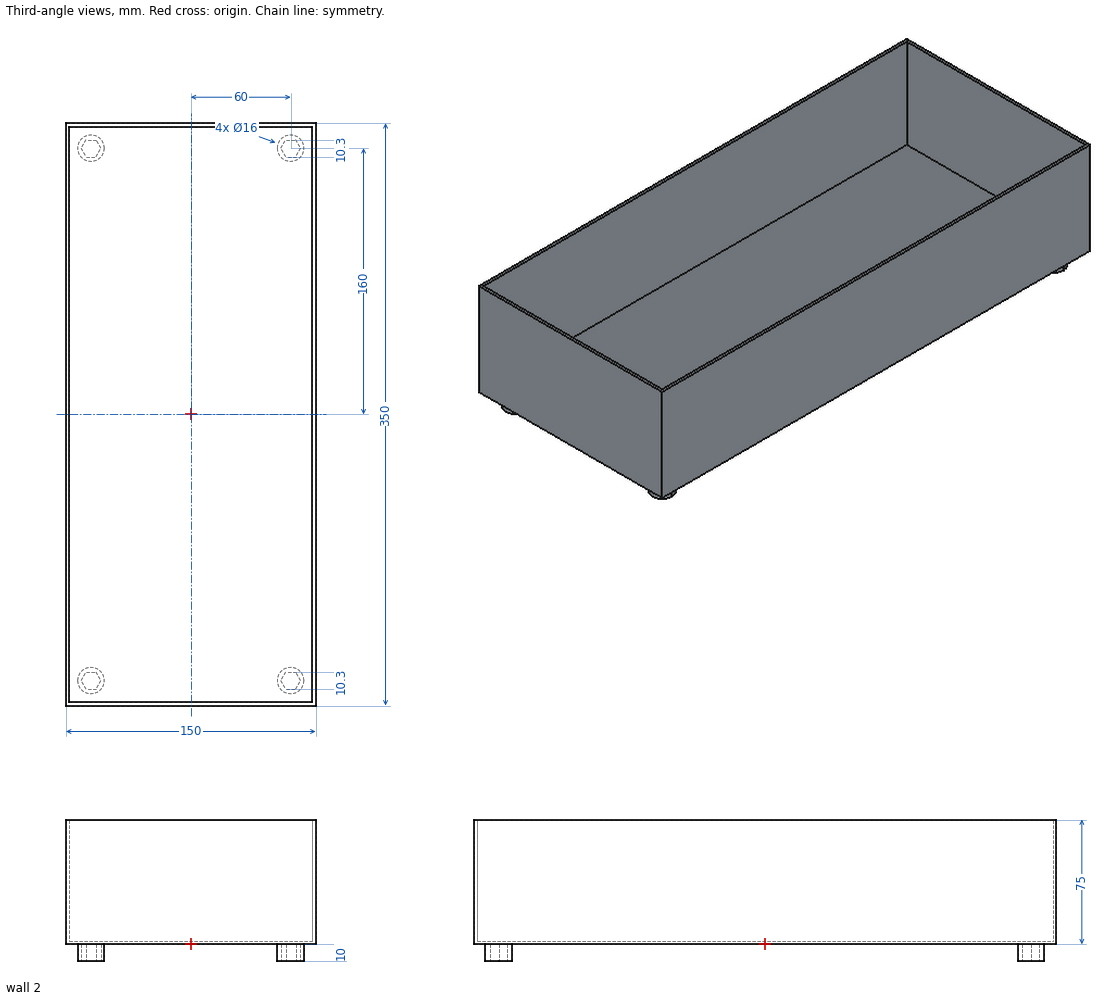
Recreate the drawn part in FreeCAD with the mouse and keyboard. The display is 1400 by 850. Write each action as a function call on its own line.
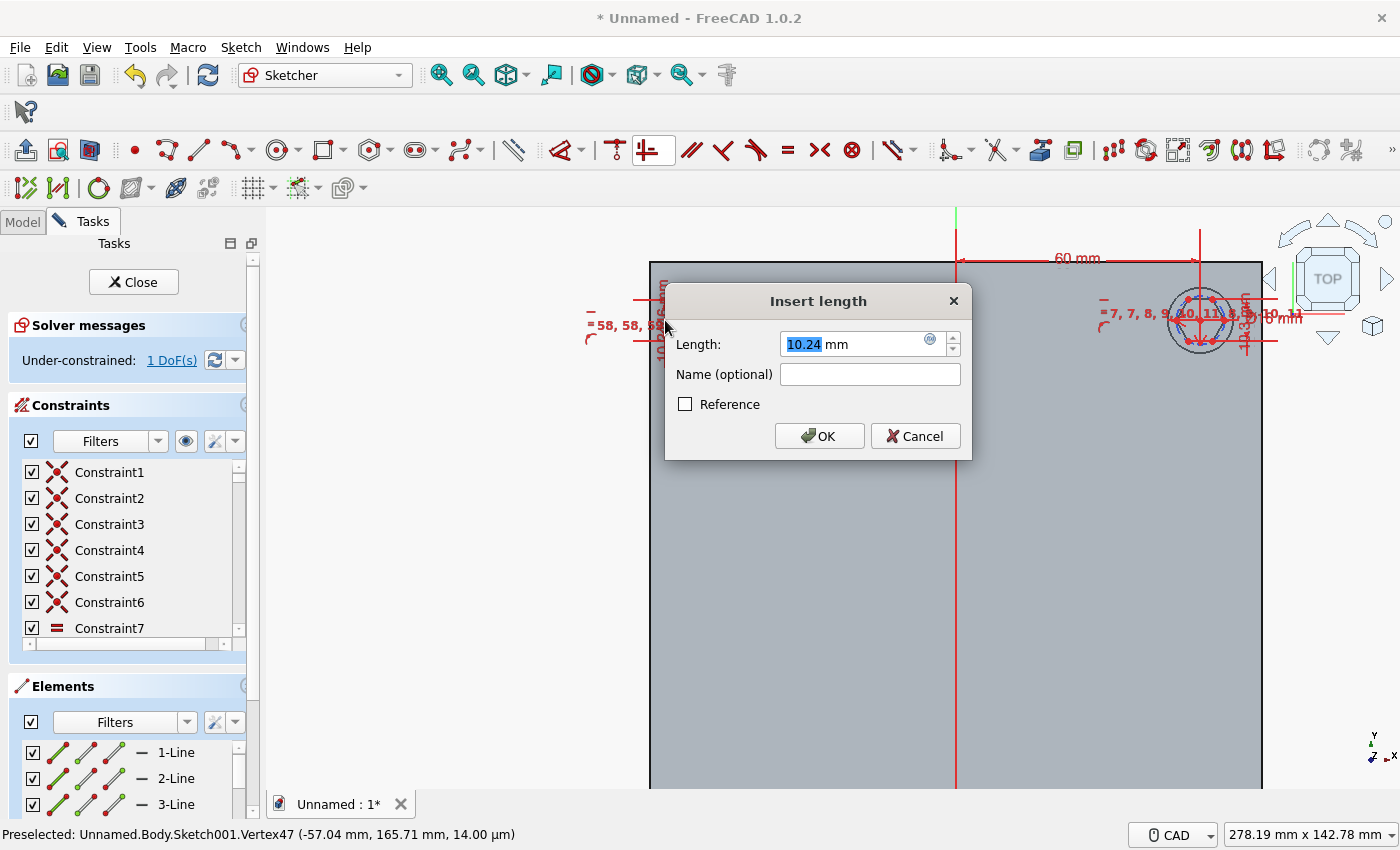
text(10.3)
key(Return)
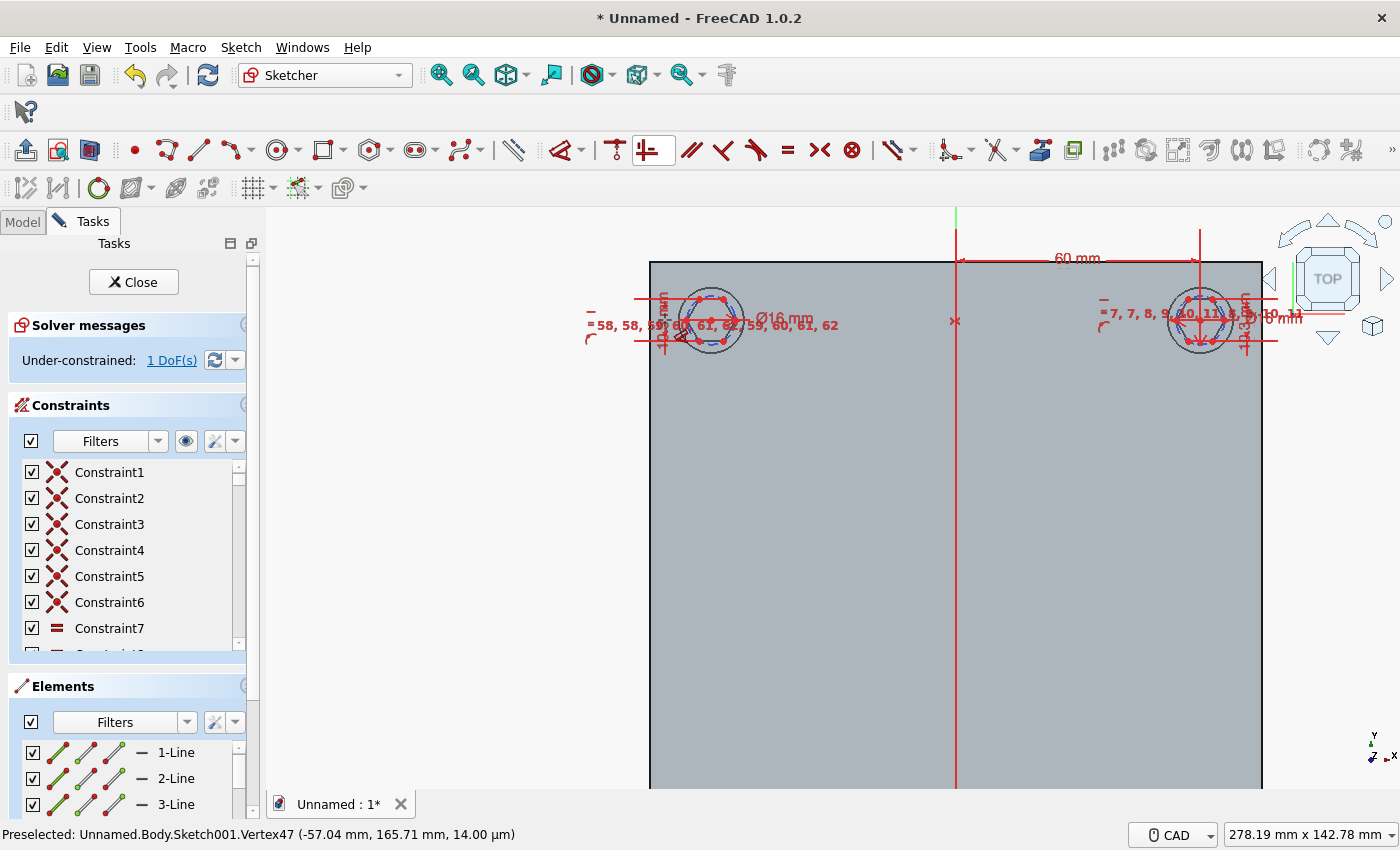
click(1200, 320)
click(1234, 541)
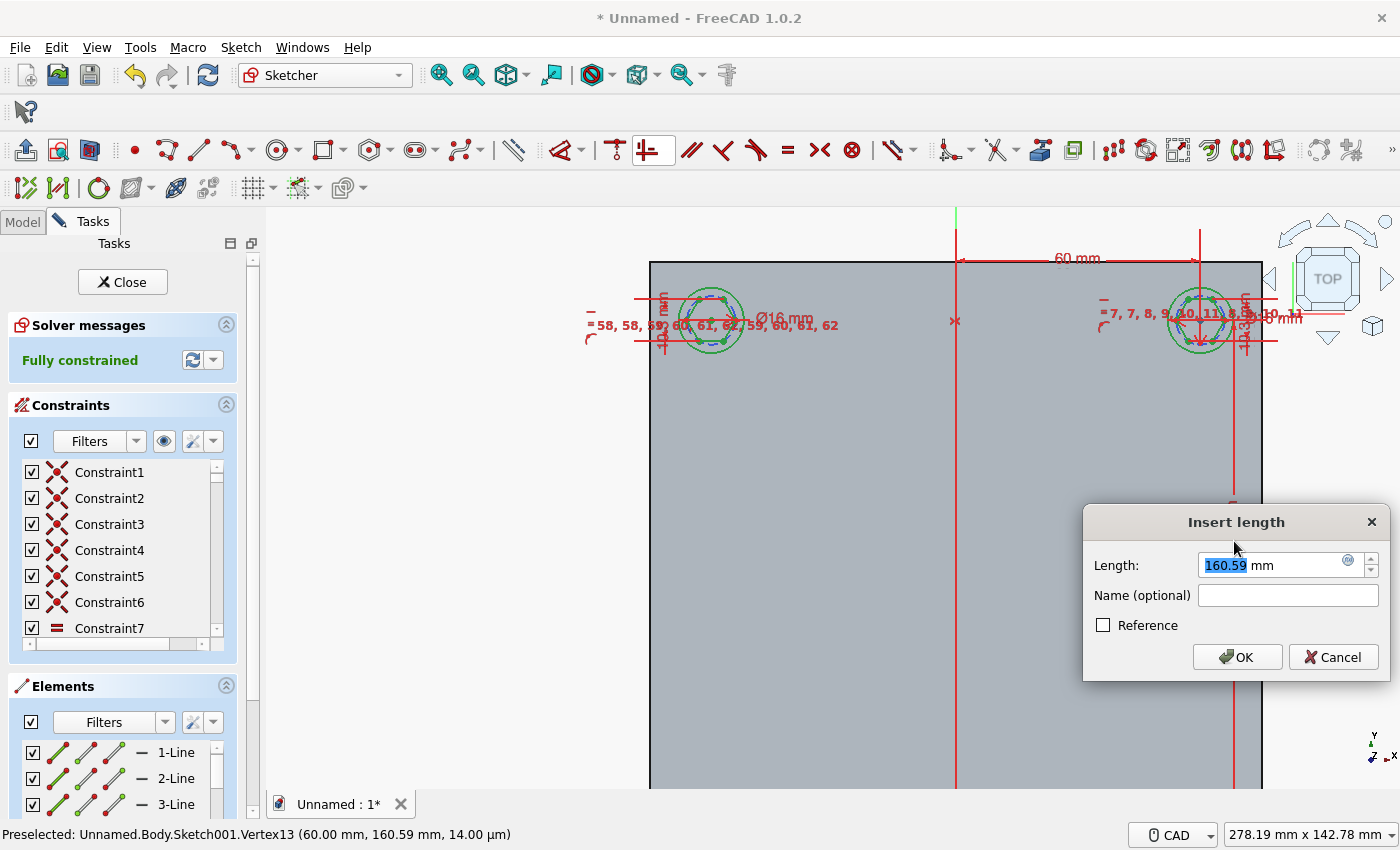
text(160)
key(Return)
key(Escape)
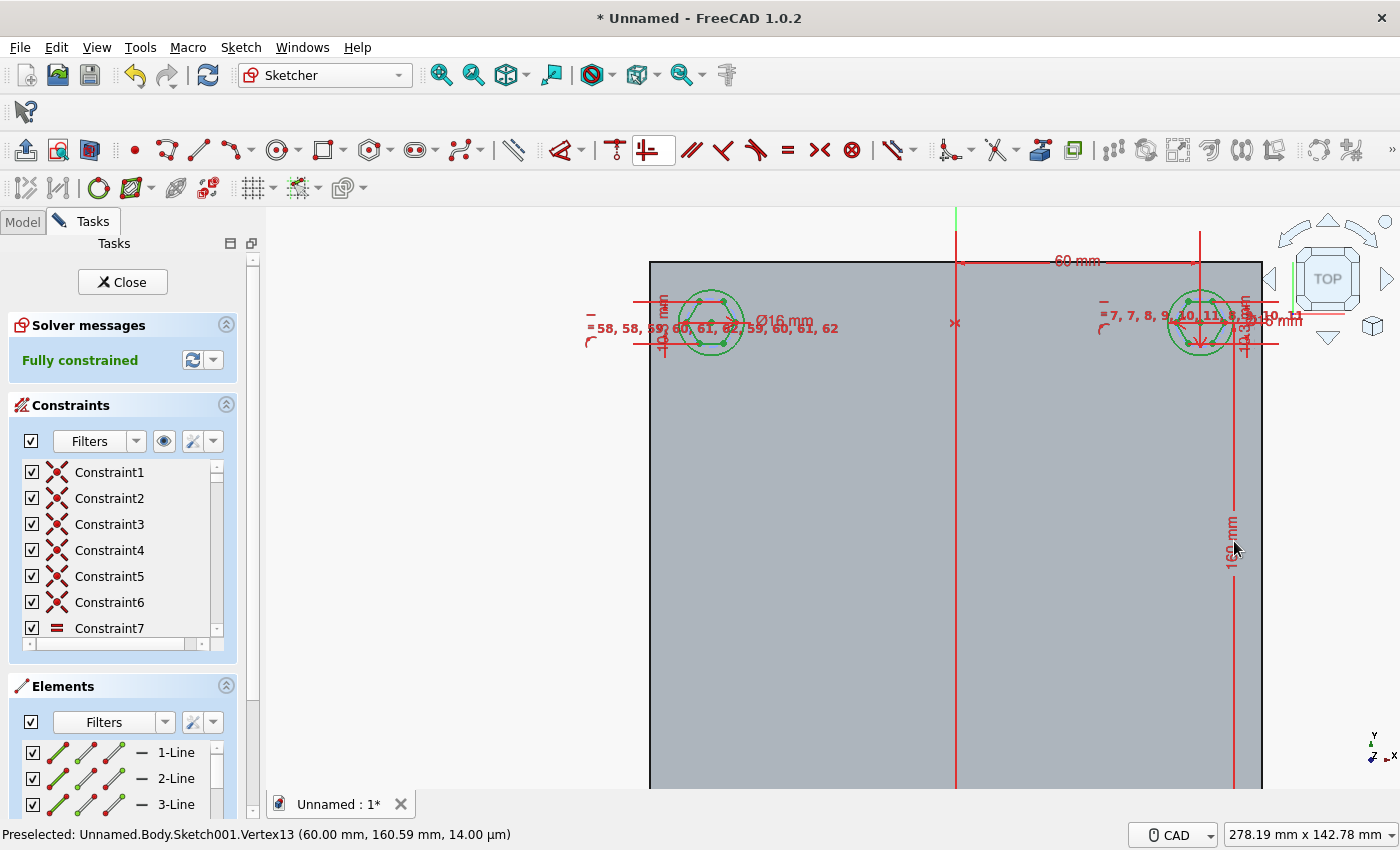
click(123, 282)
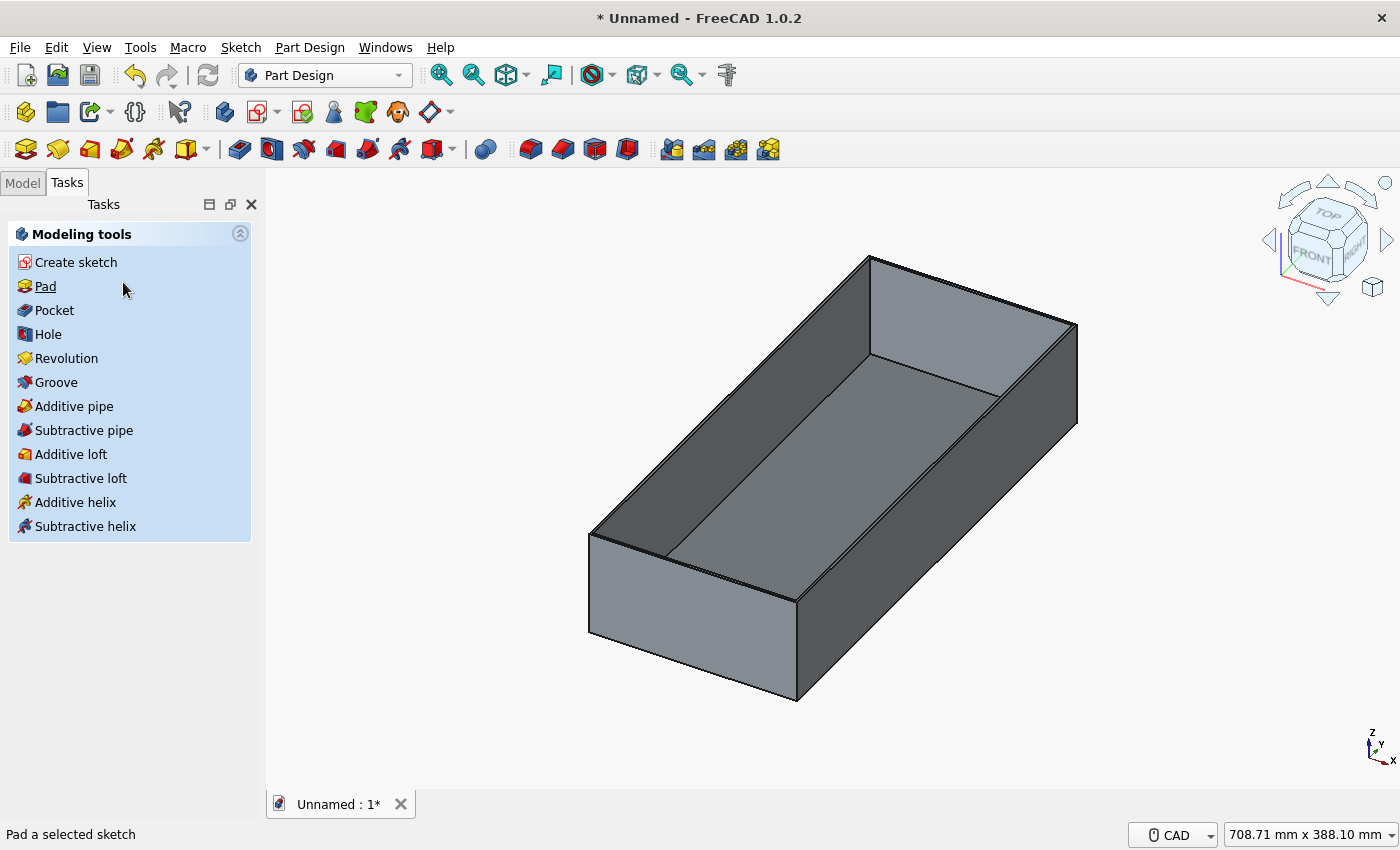
click(26, 150)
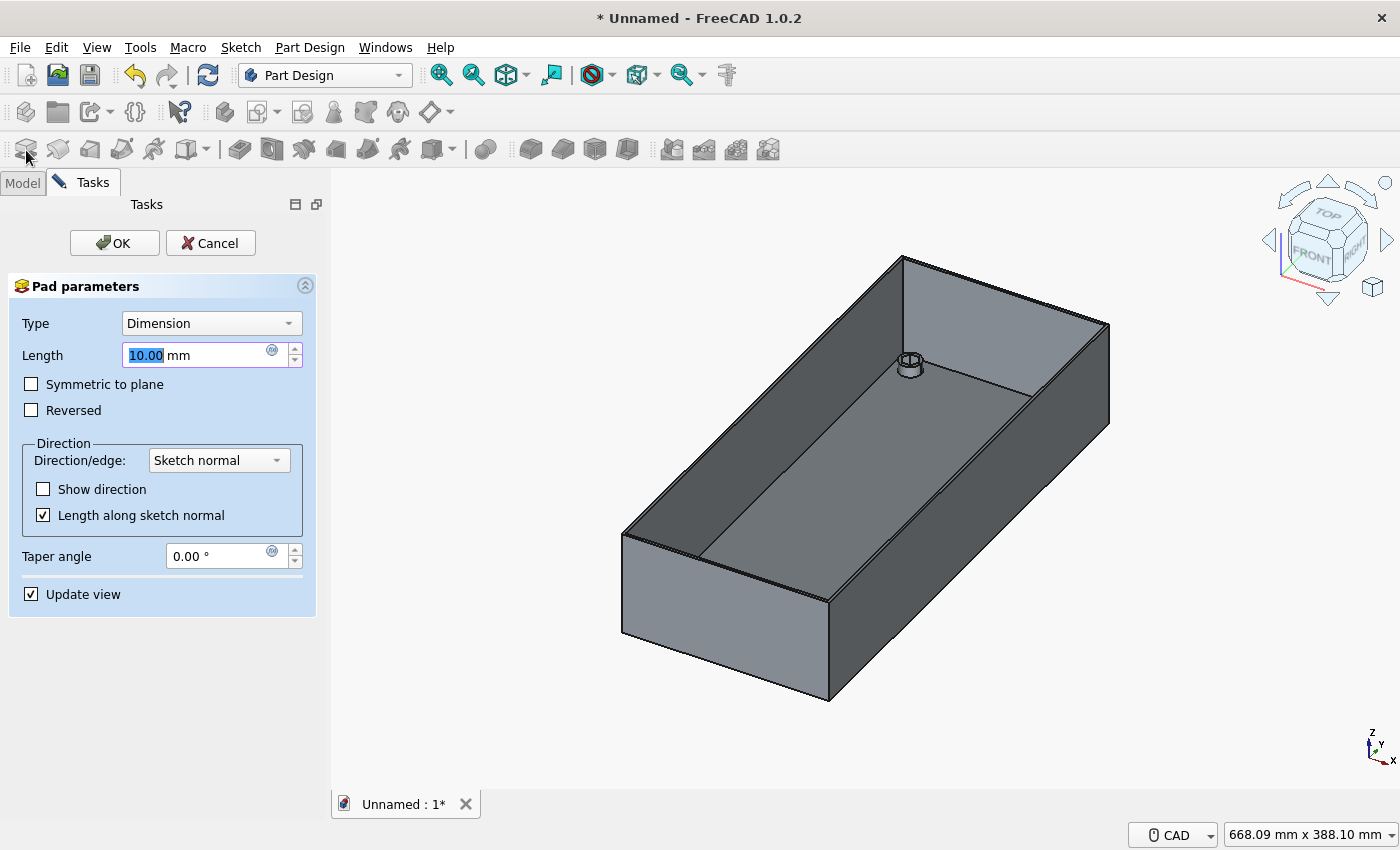
text(10)
key(Tab)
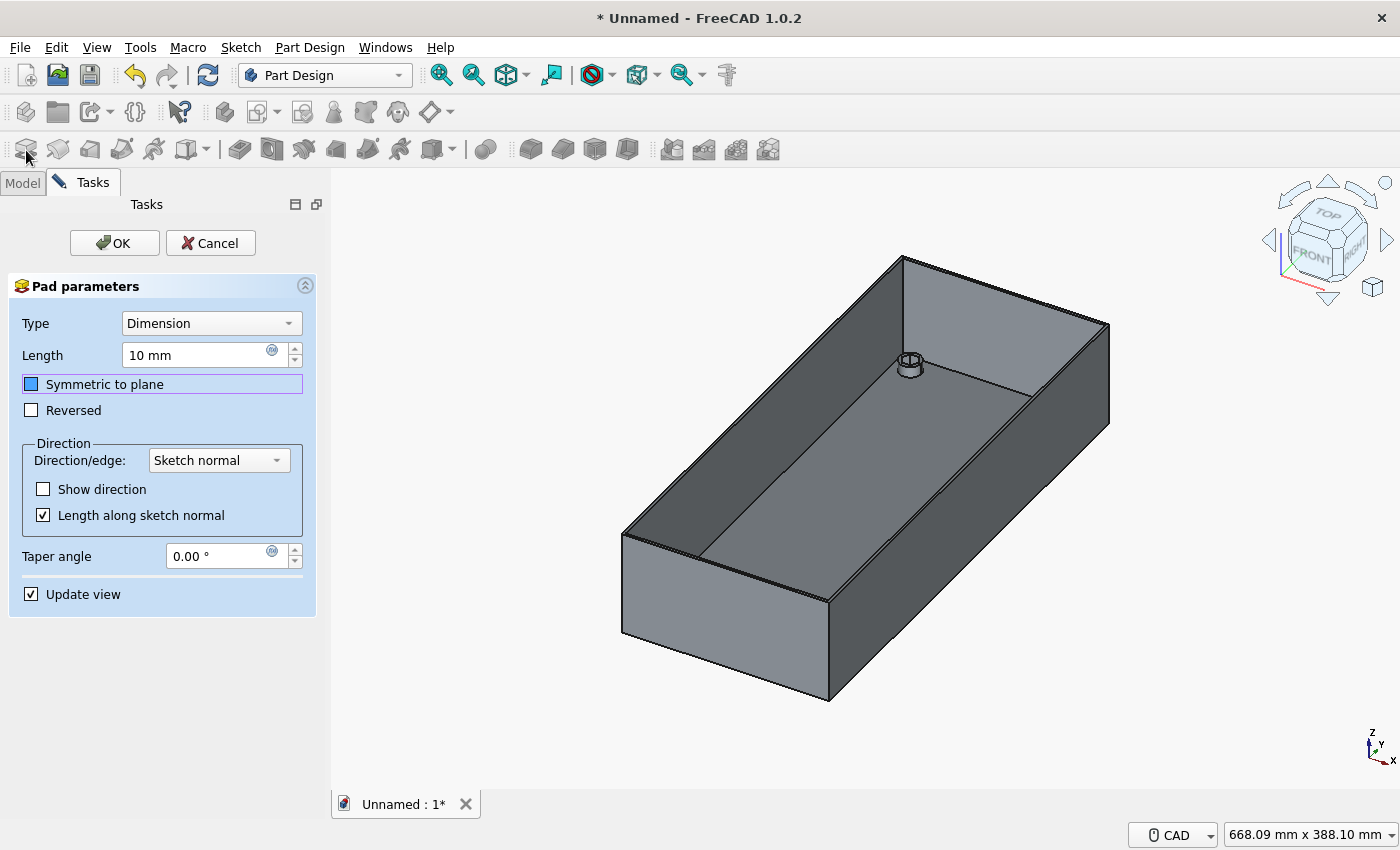
click(30, 410)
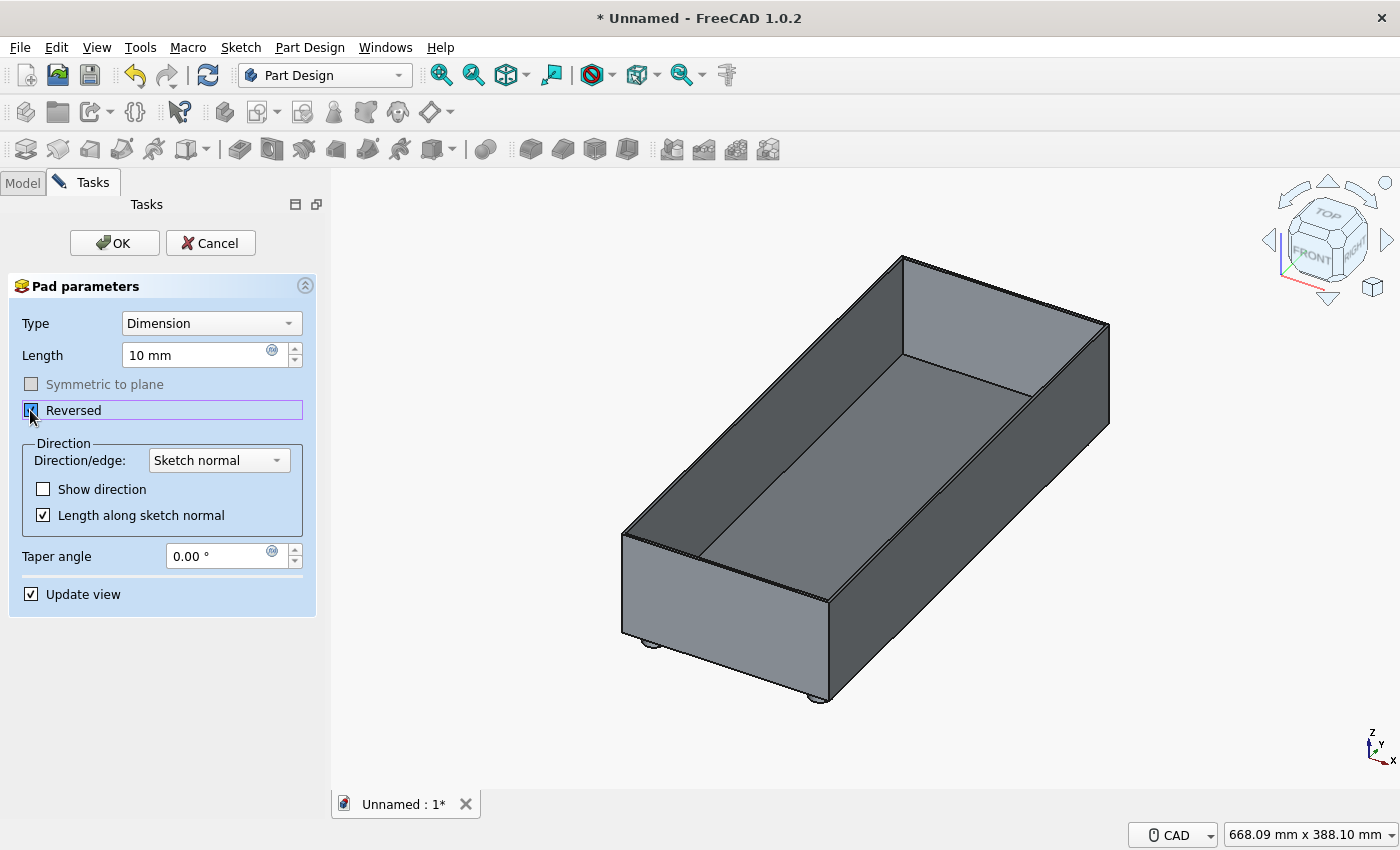
click(115, 243)